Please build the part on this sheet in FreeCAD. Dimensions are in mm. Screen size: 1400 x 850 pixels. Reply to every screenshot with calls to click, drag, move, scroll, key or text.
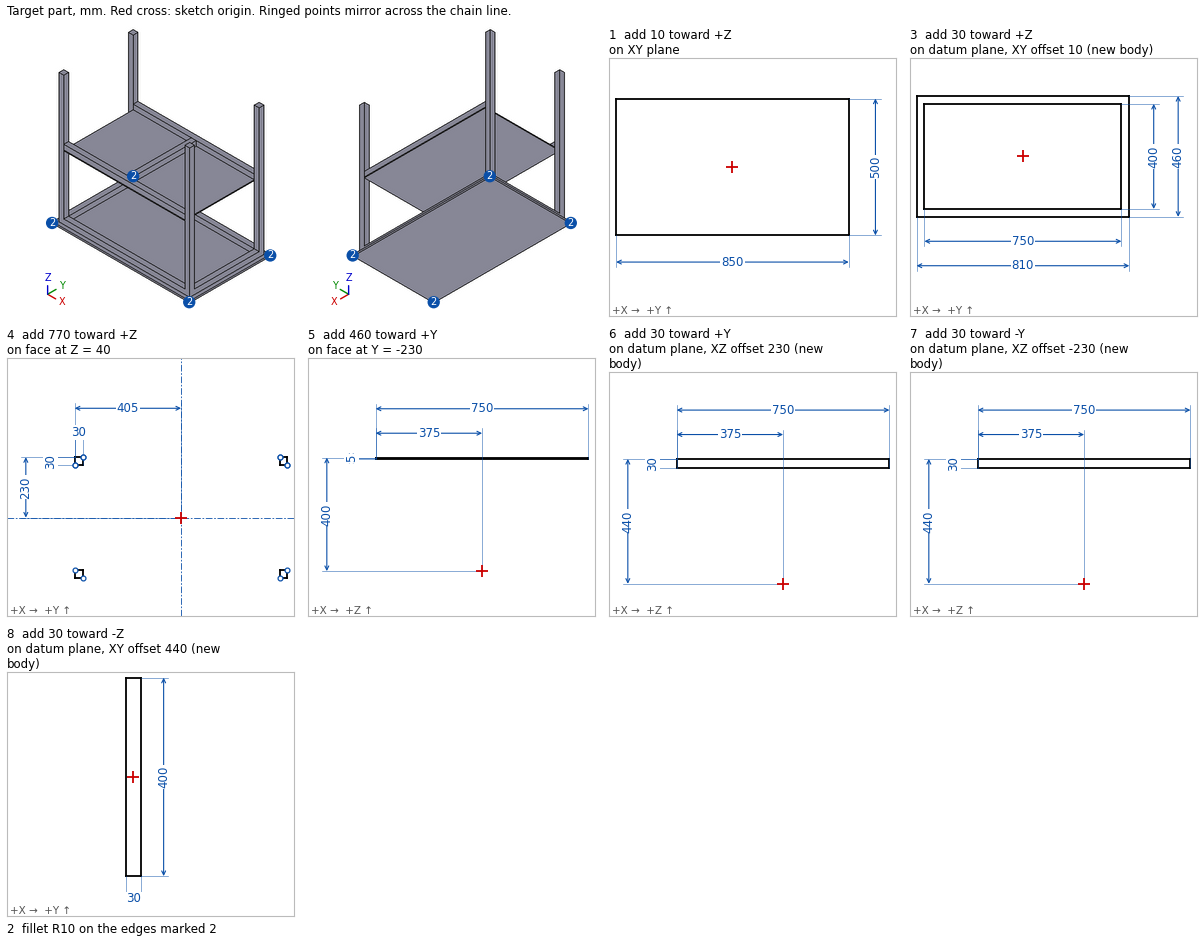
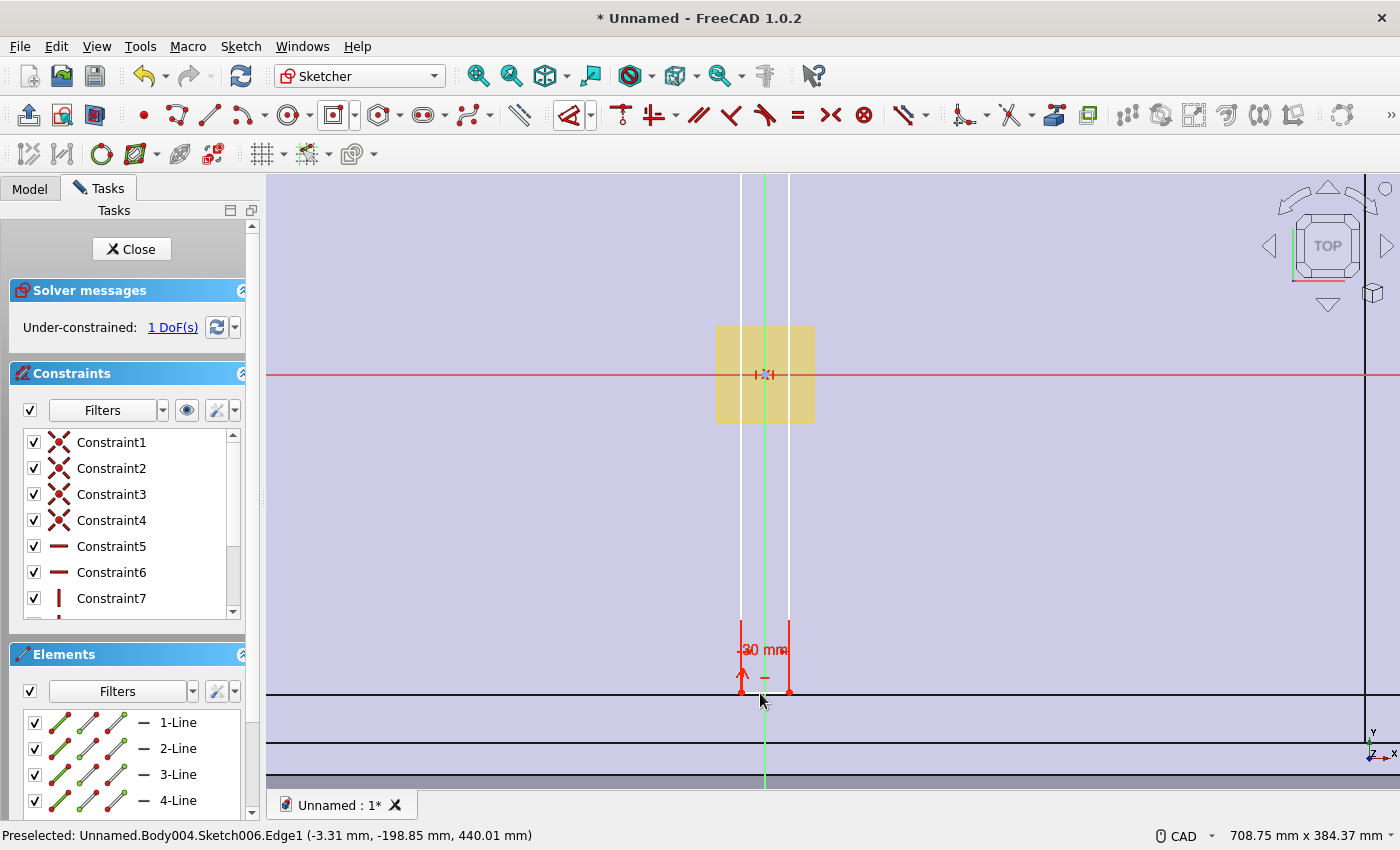
click(789, 502)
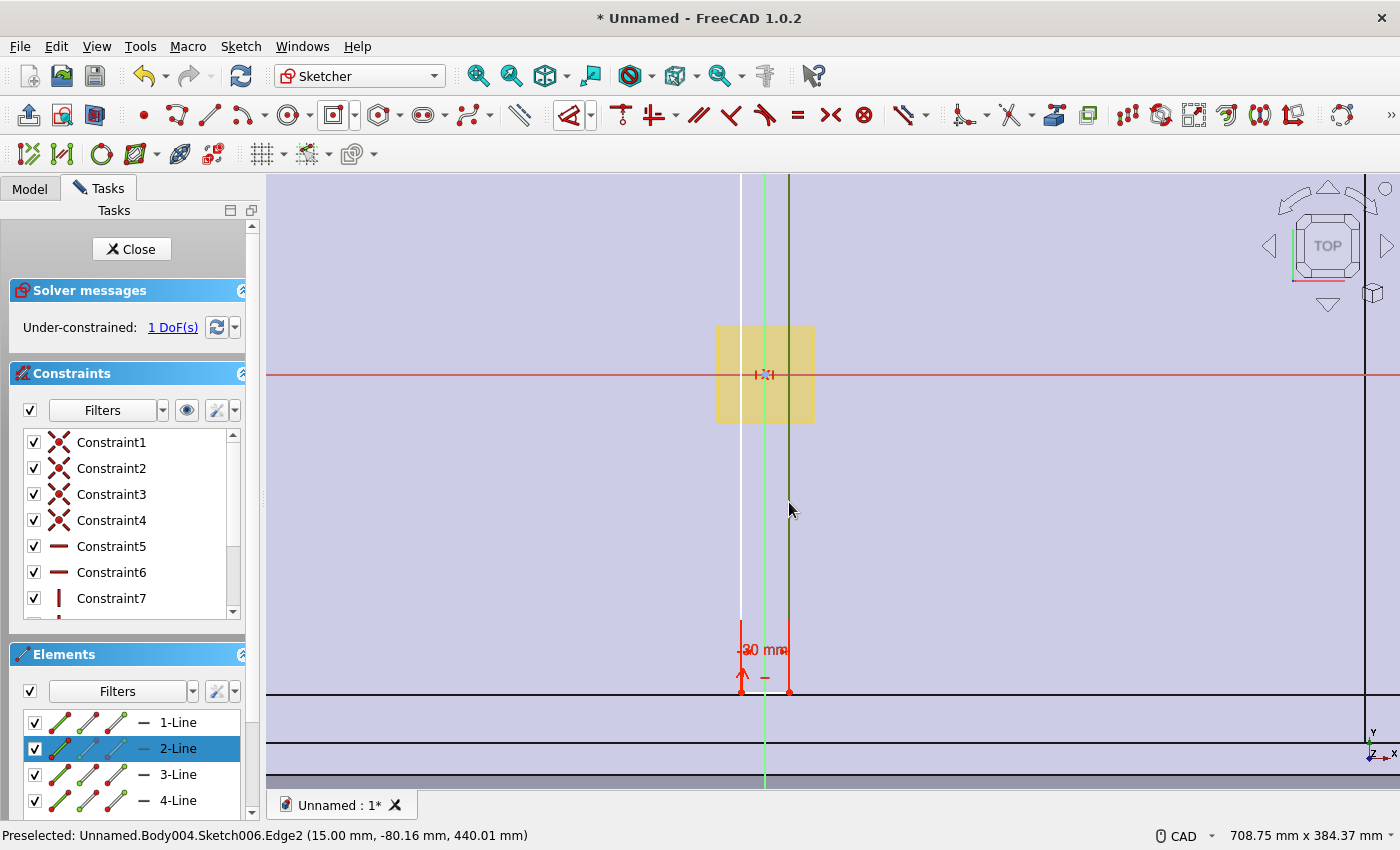
click(590, 116)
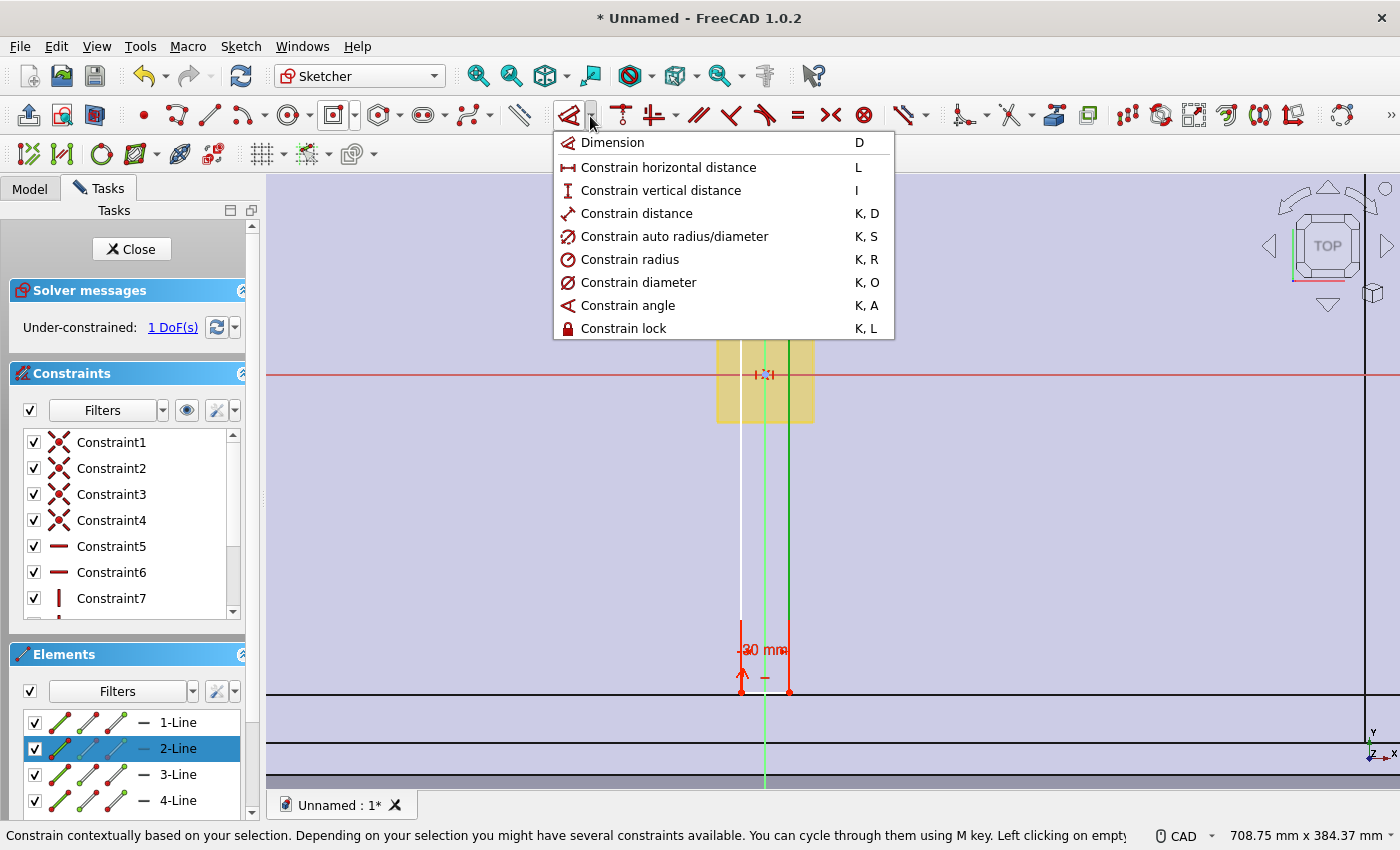
click(724, 190)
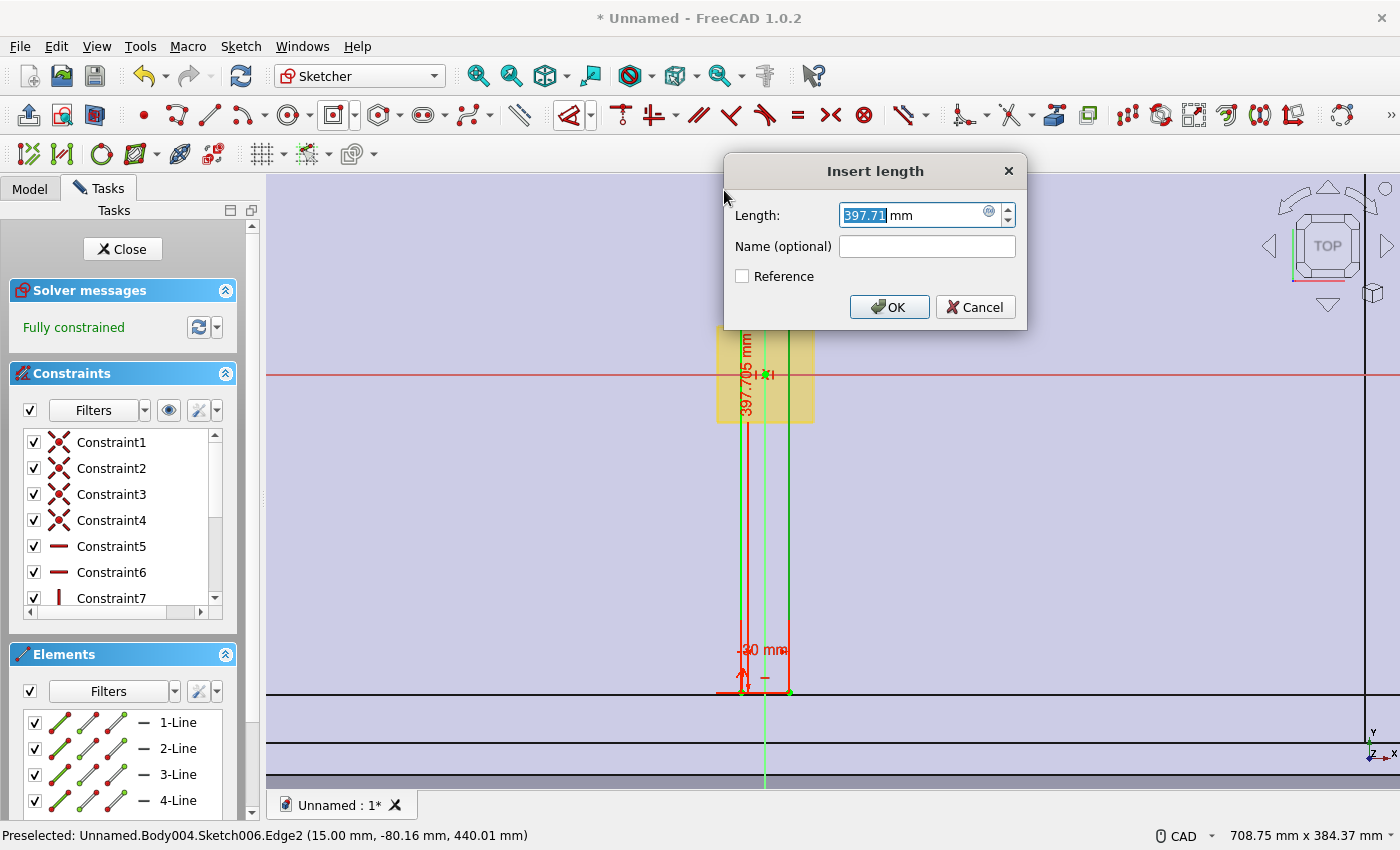
text(400)
key(Return)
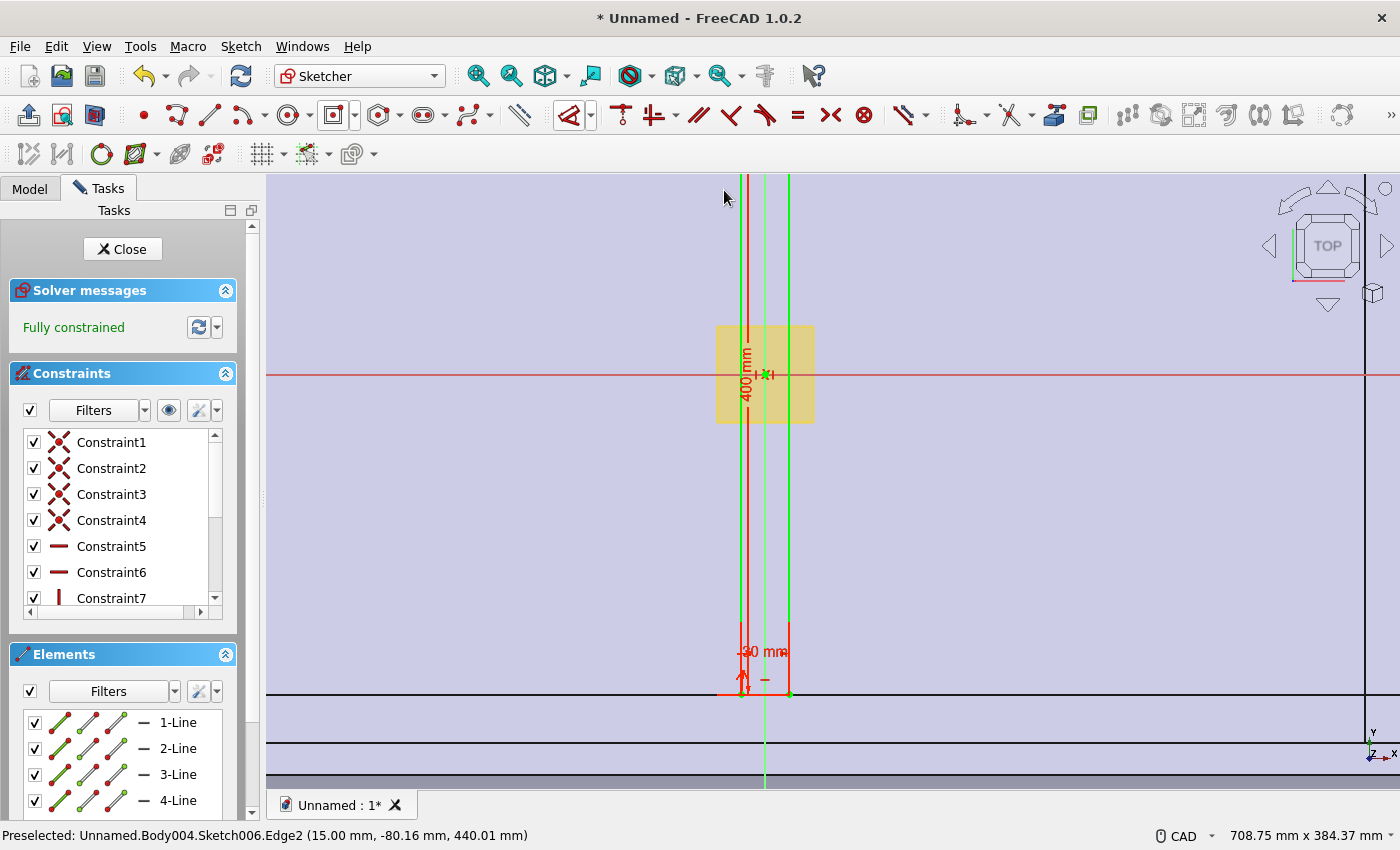
click(123, 249)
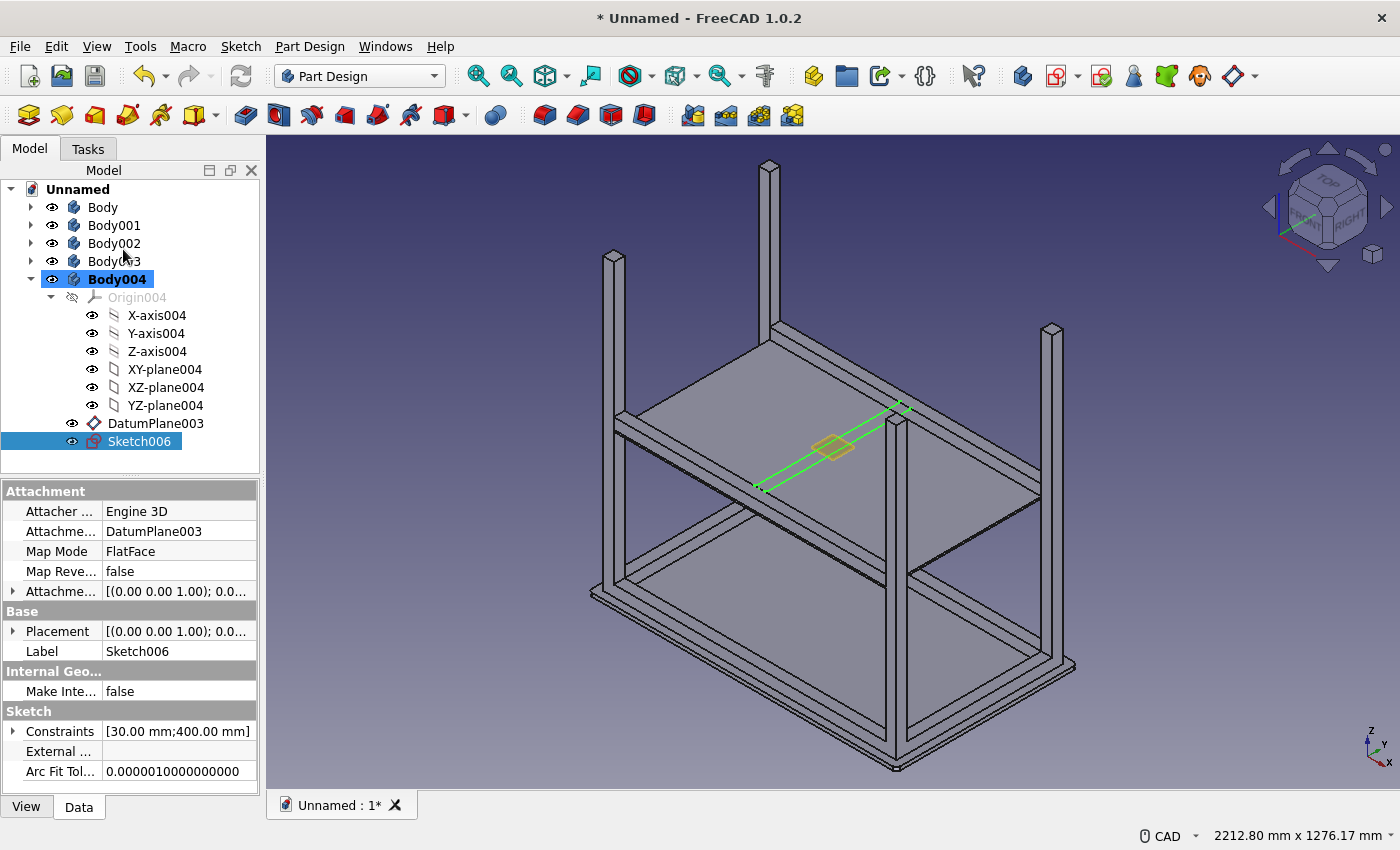
click(29, 116)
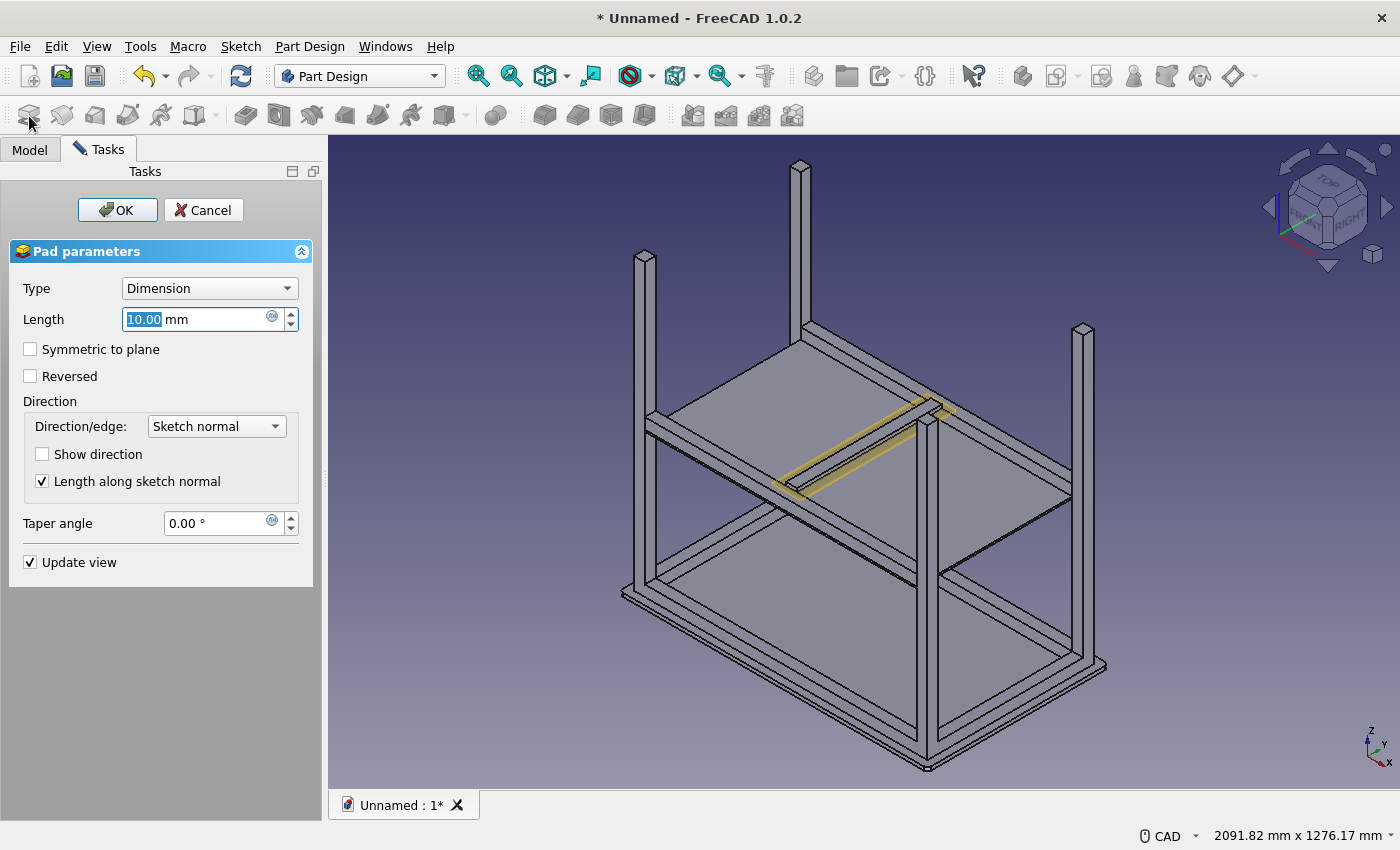
text(30)
key(Tab)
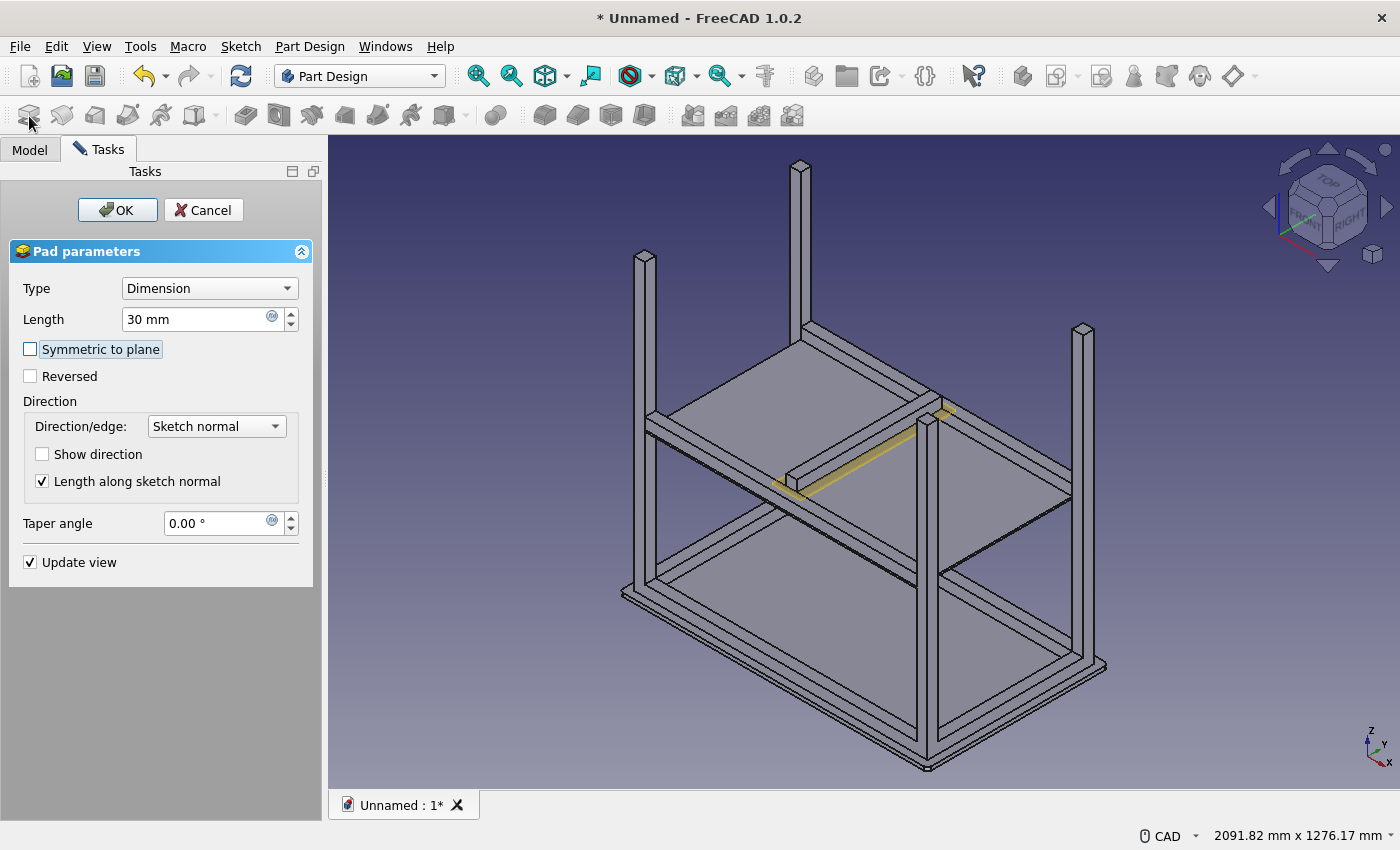
click(31, 376)